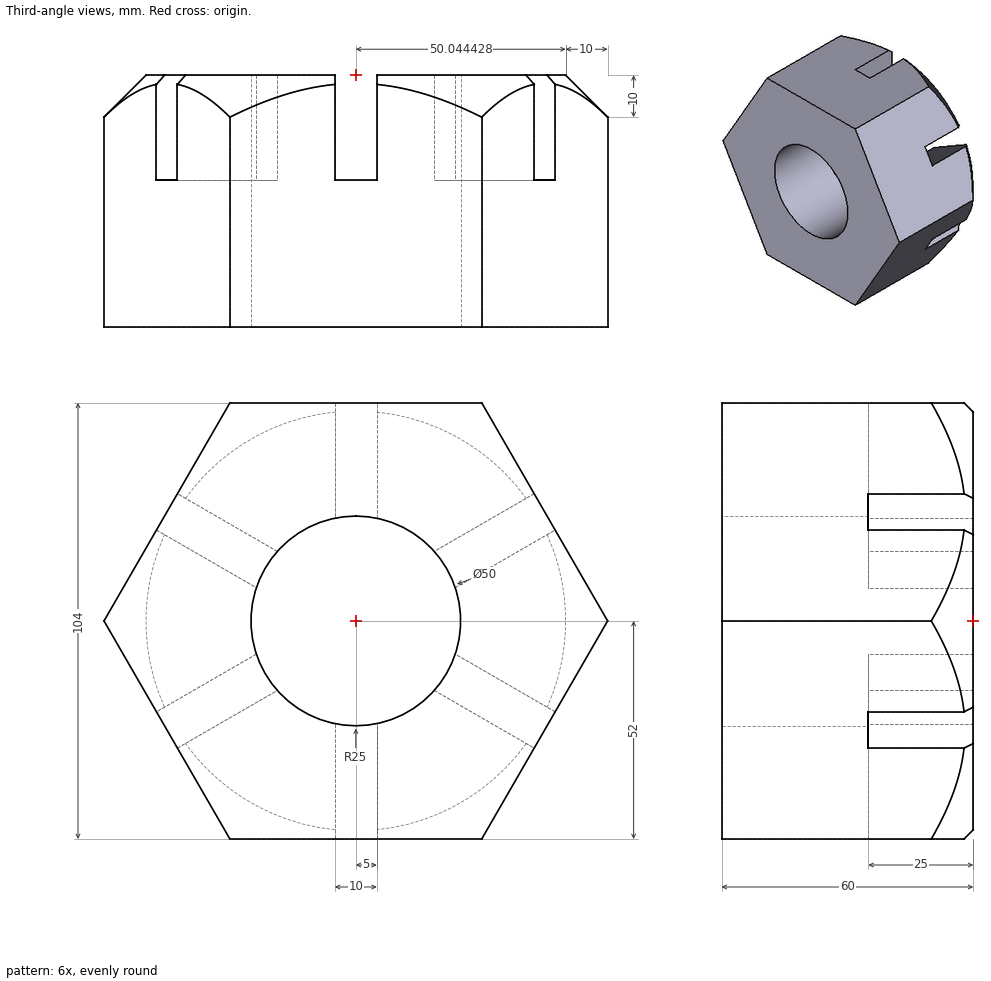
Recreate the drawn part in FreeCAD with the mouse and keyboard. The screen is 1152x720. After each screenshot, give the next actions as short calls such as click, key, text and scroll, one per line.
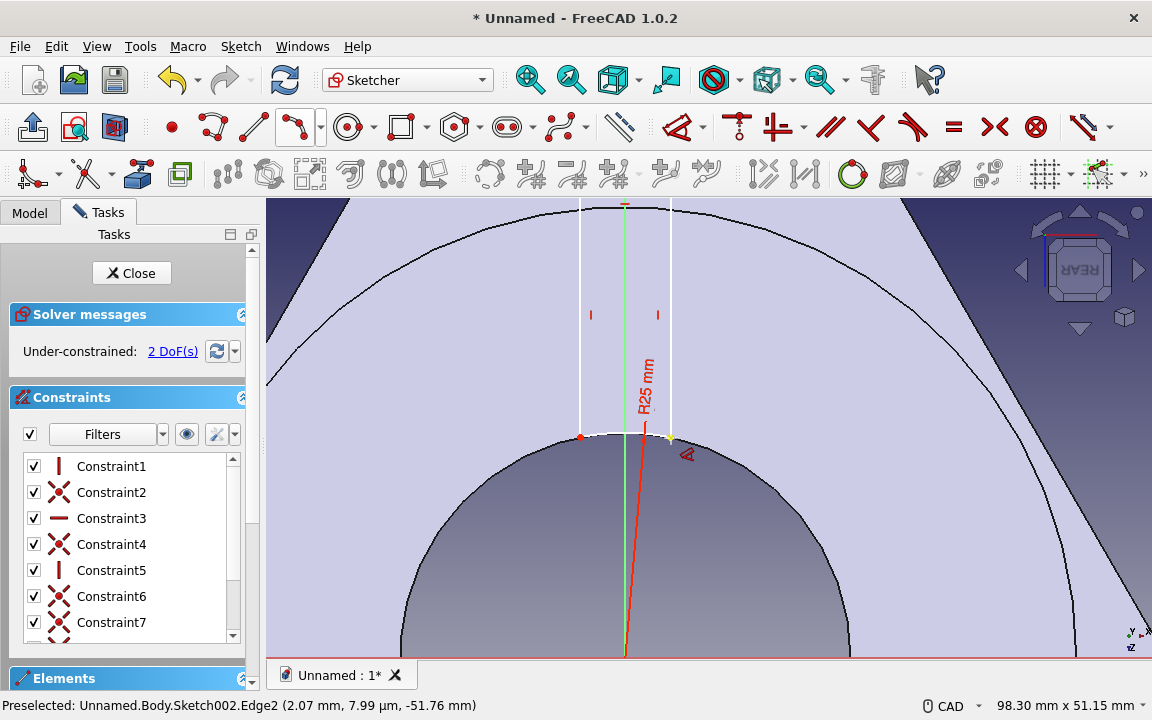
click(671, 437)
click(648, 355)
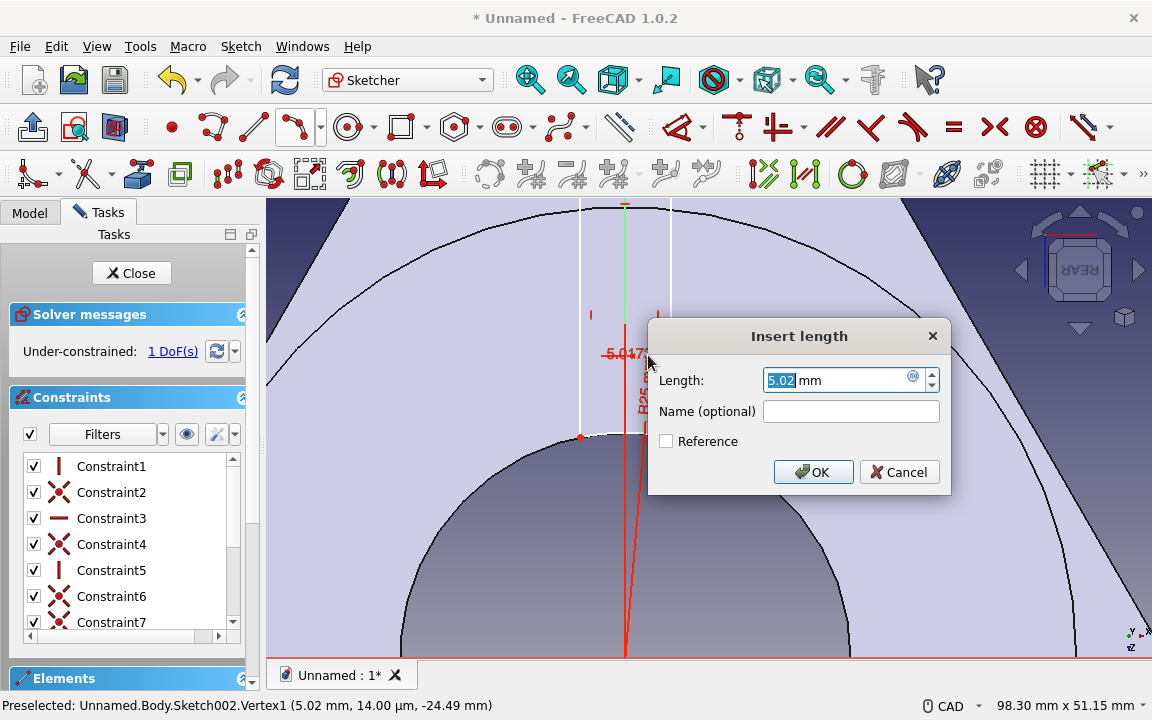
text(5)
key(Return)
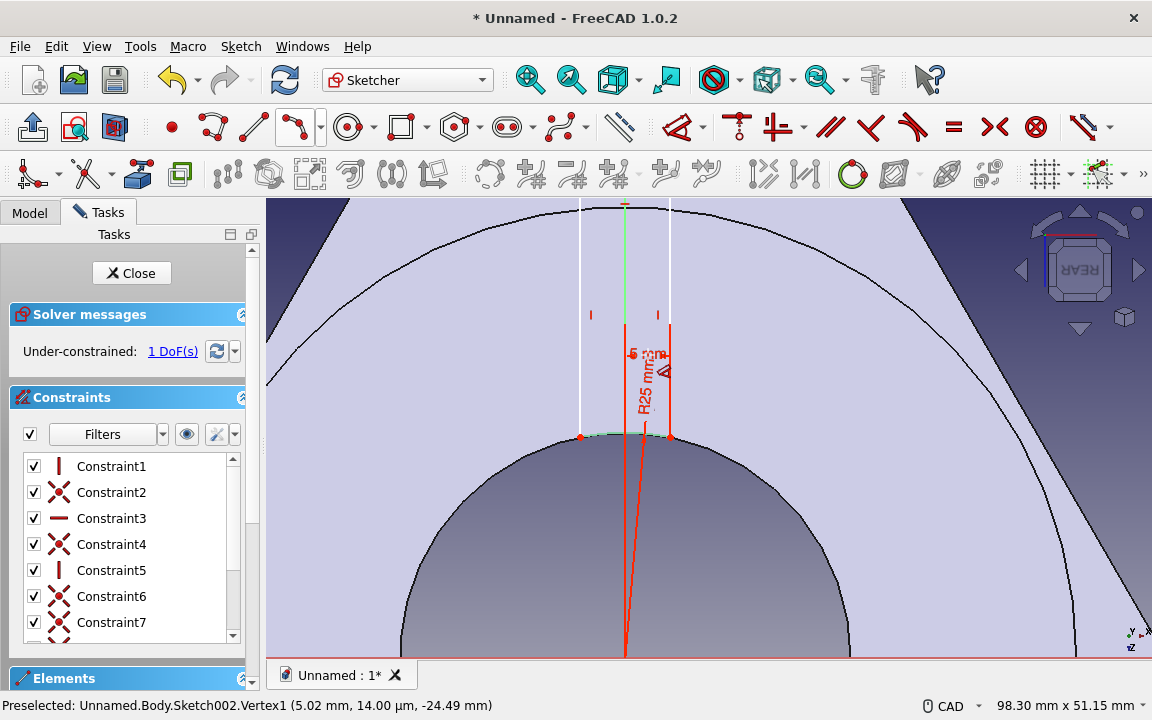
scroll(671, 438, down, 2)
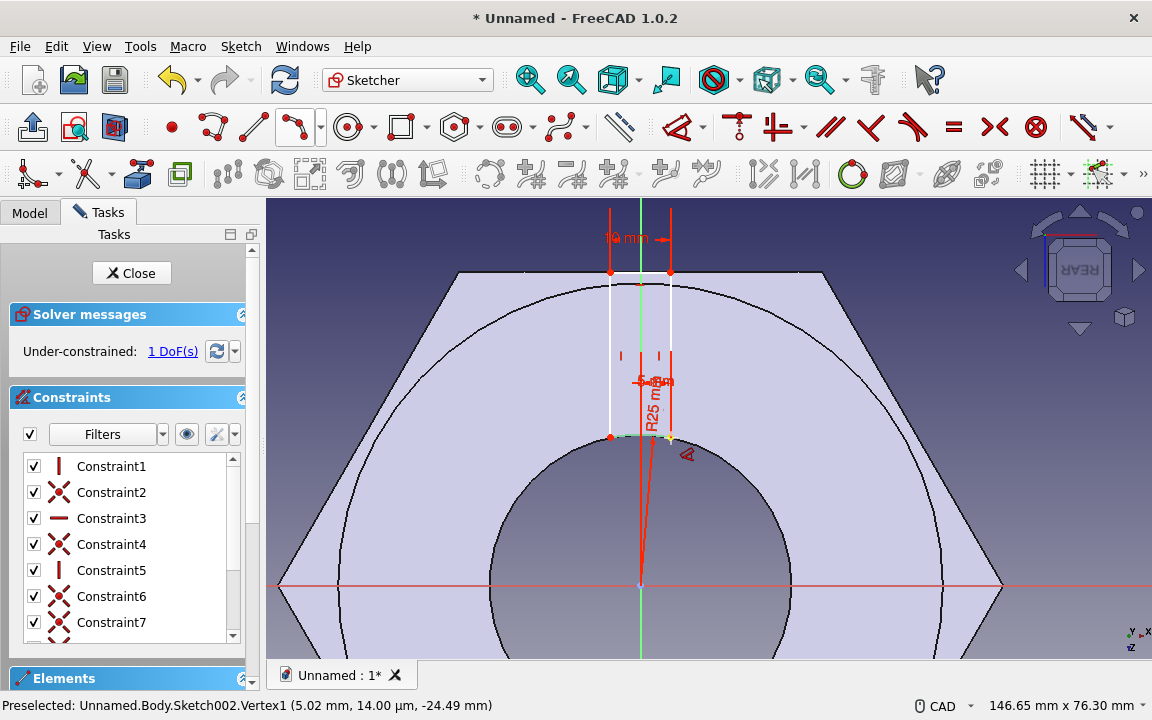
click(671, 273)
click(705, 429)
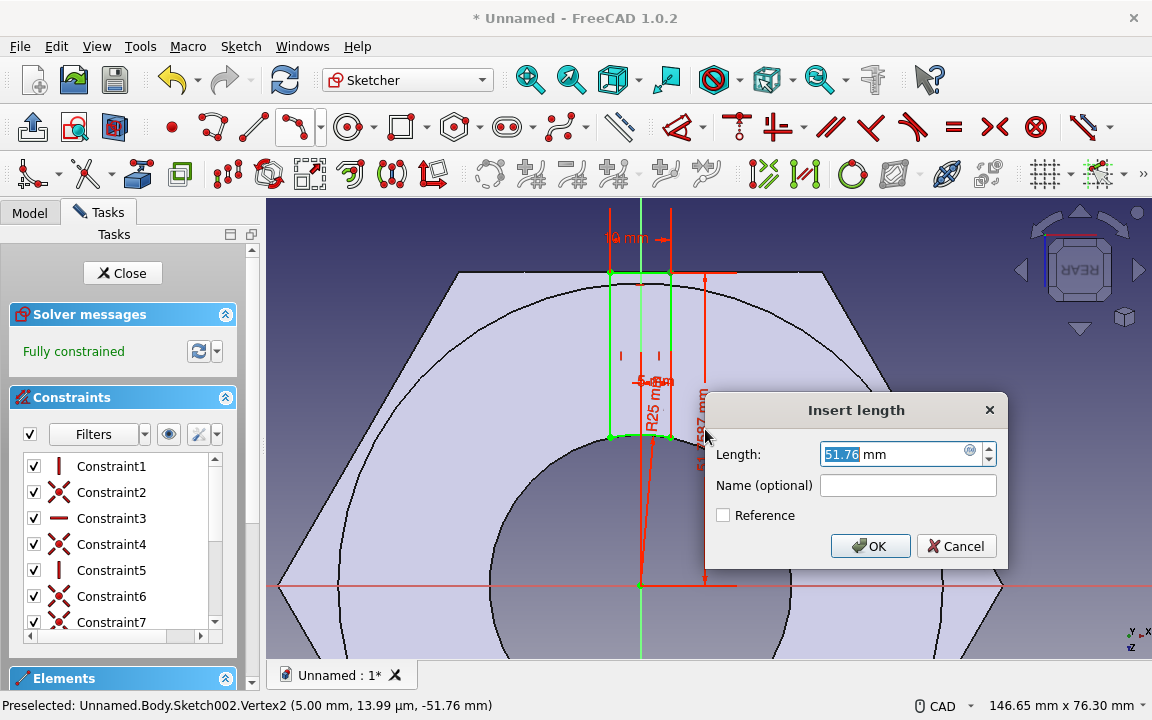
text(52)
key(Return)
key(Escape)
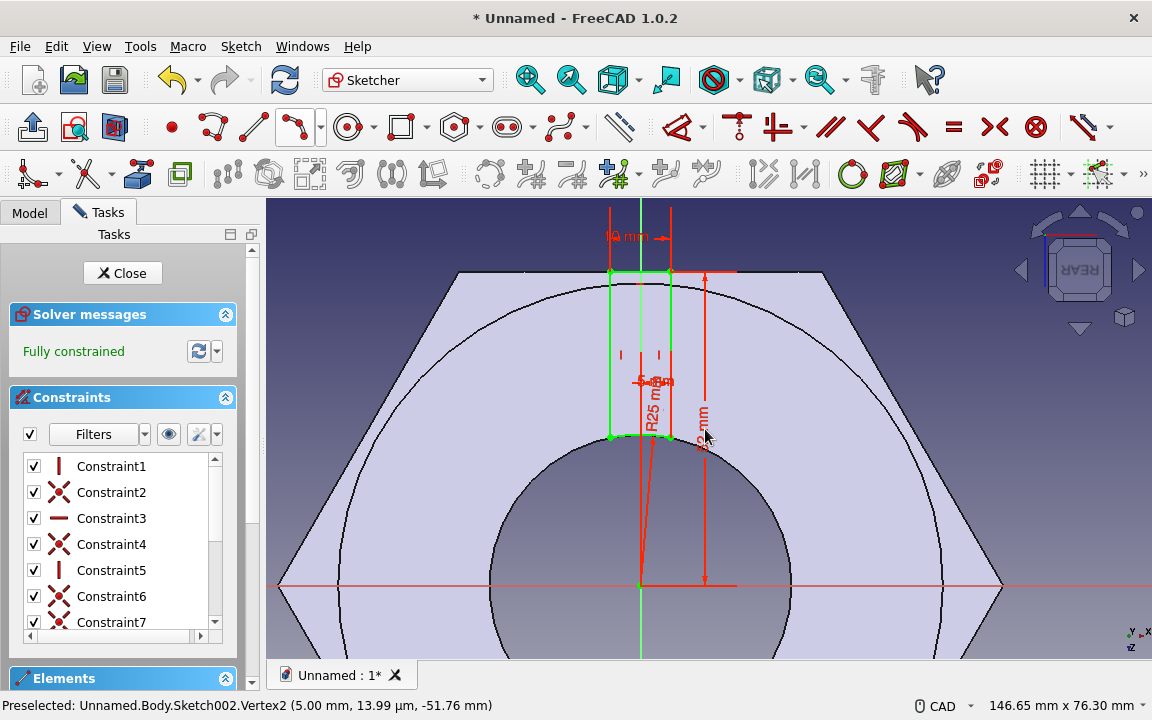
click(123, 273)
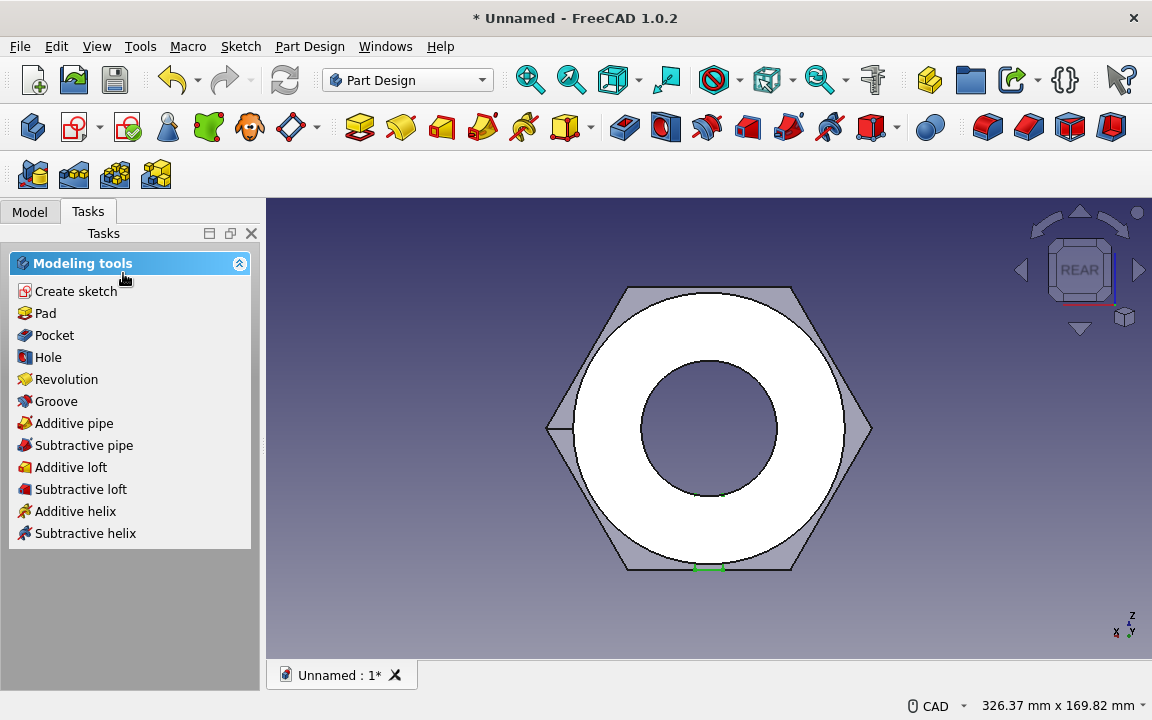
click(625, 128)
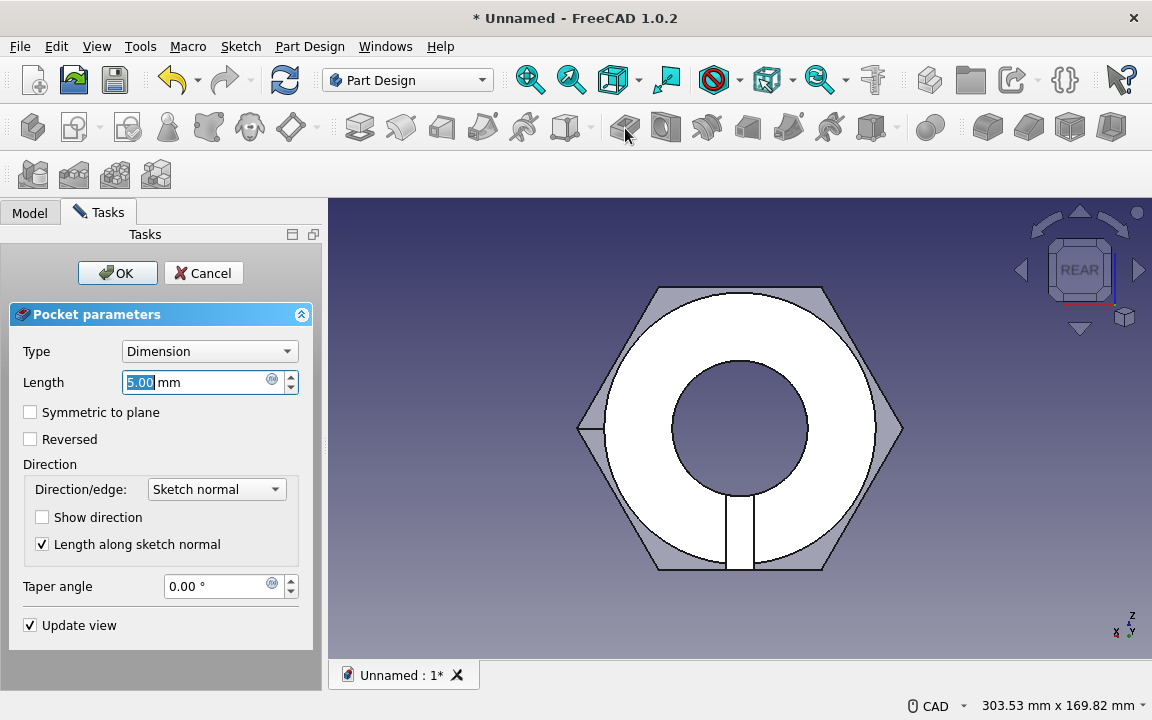
text(25)
key(Tab)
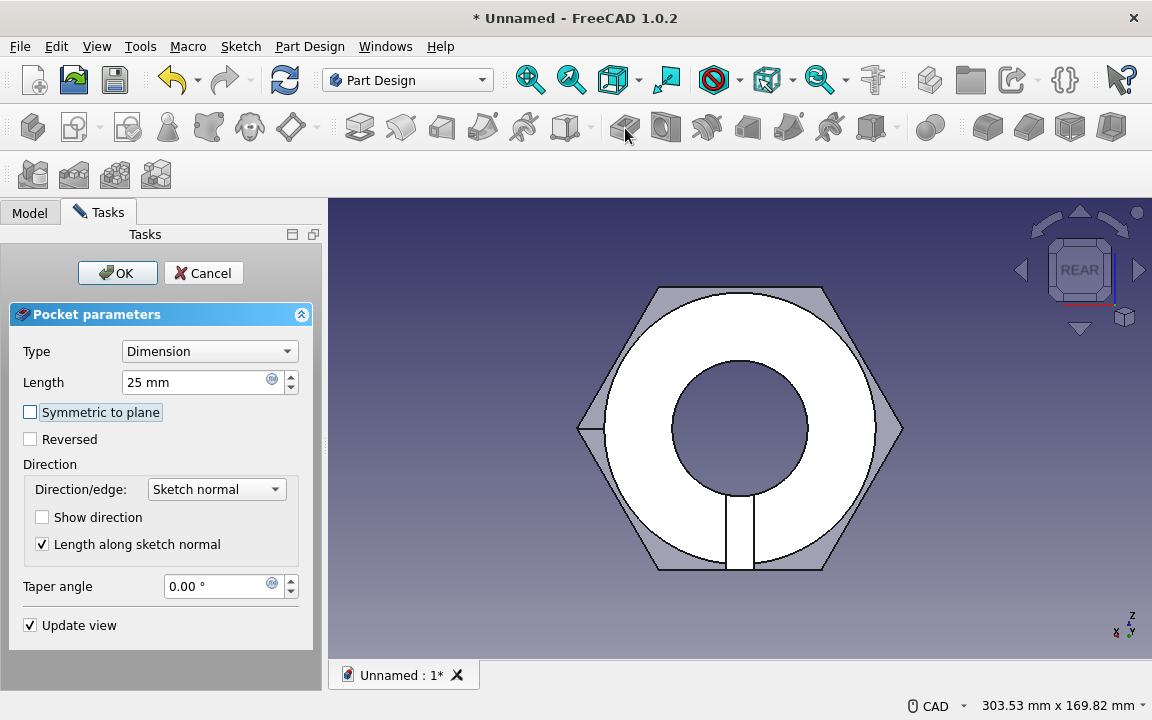
click(118, 273)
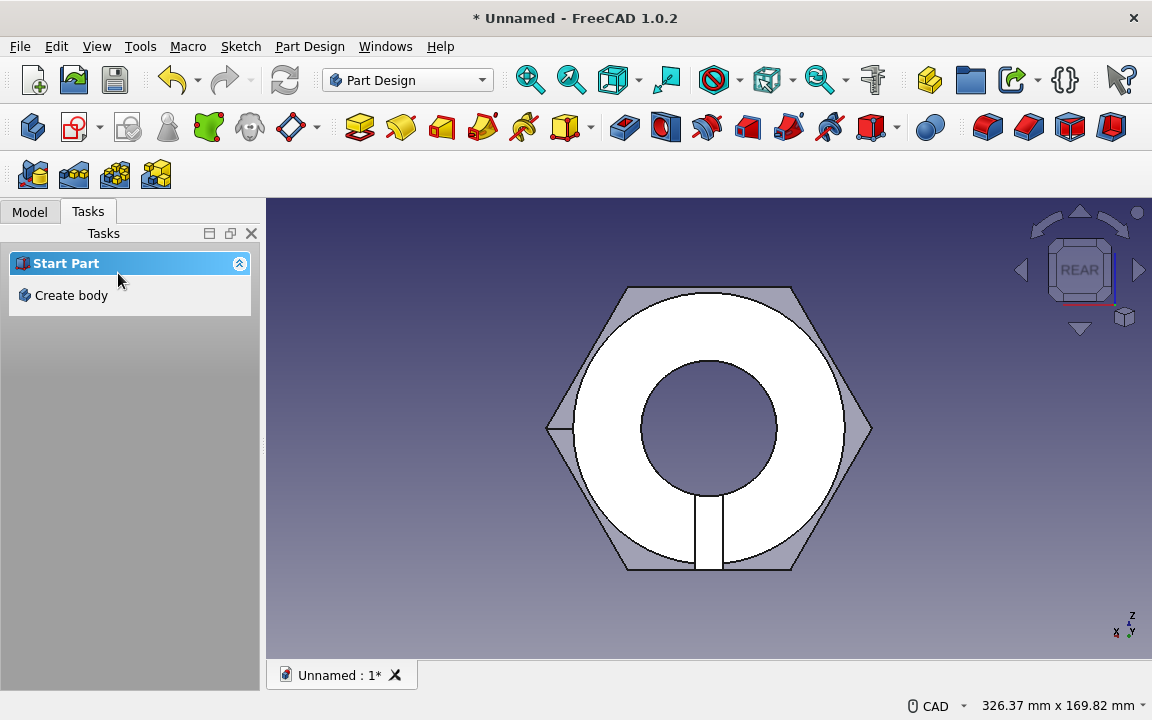
click(30, 212)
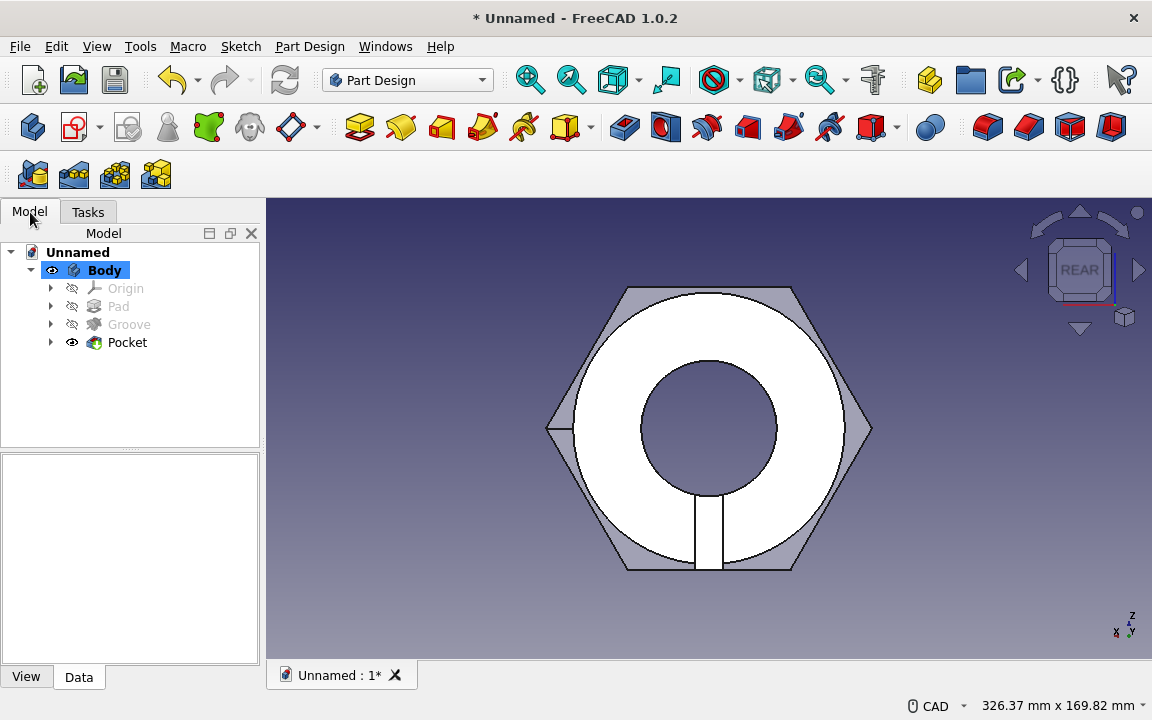
click(117, 342)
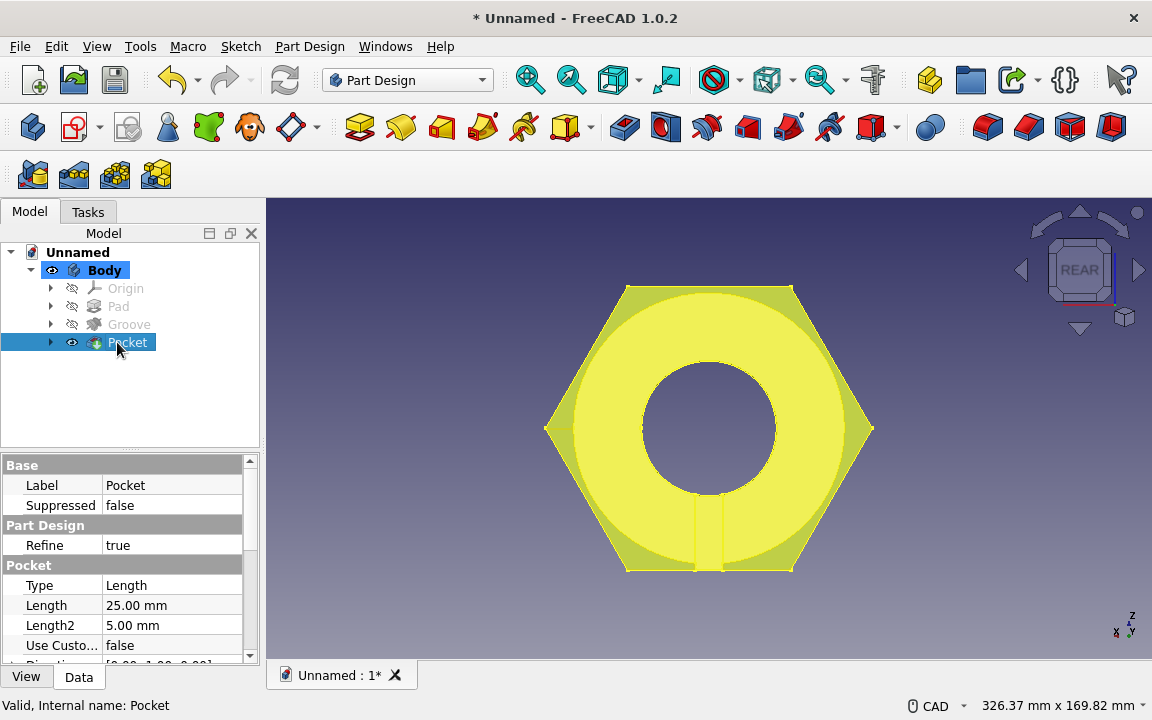
click(115, 174)